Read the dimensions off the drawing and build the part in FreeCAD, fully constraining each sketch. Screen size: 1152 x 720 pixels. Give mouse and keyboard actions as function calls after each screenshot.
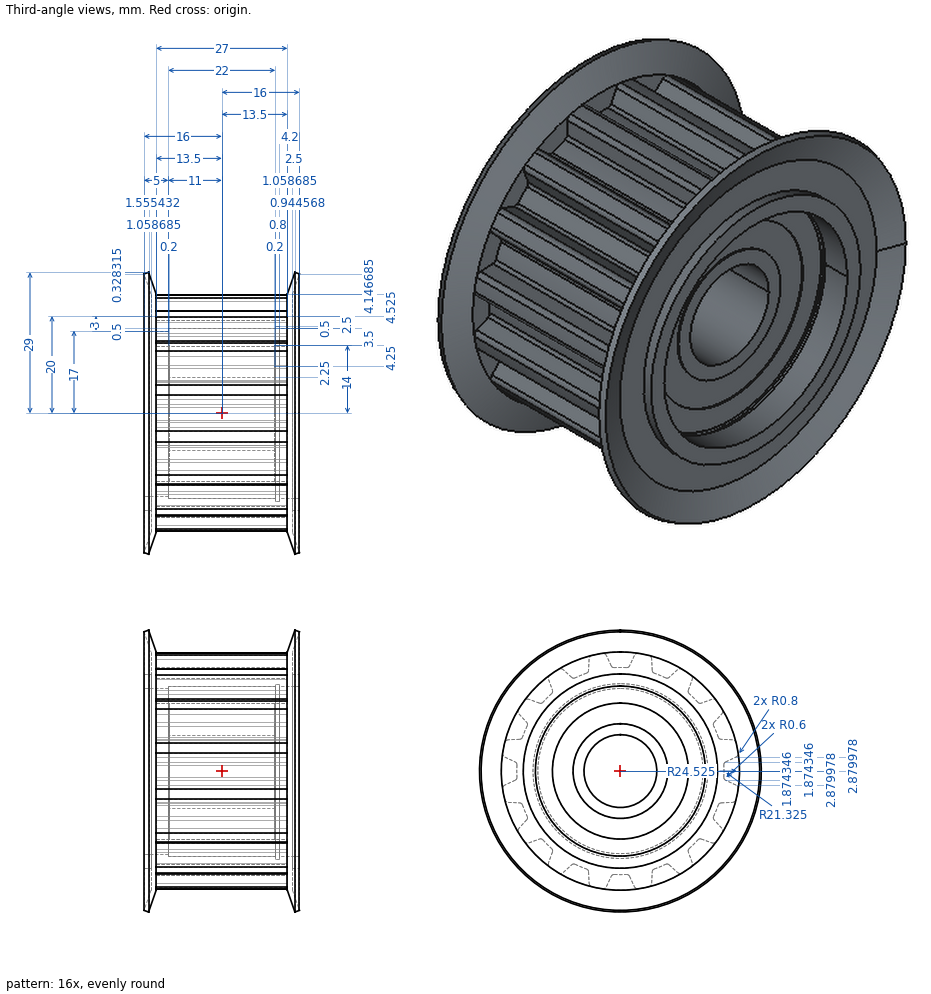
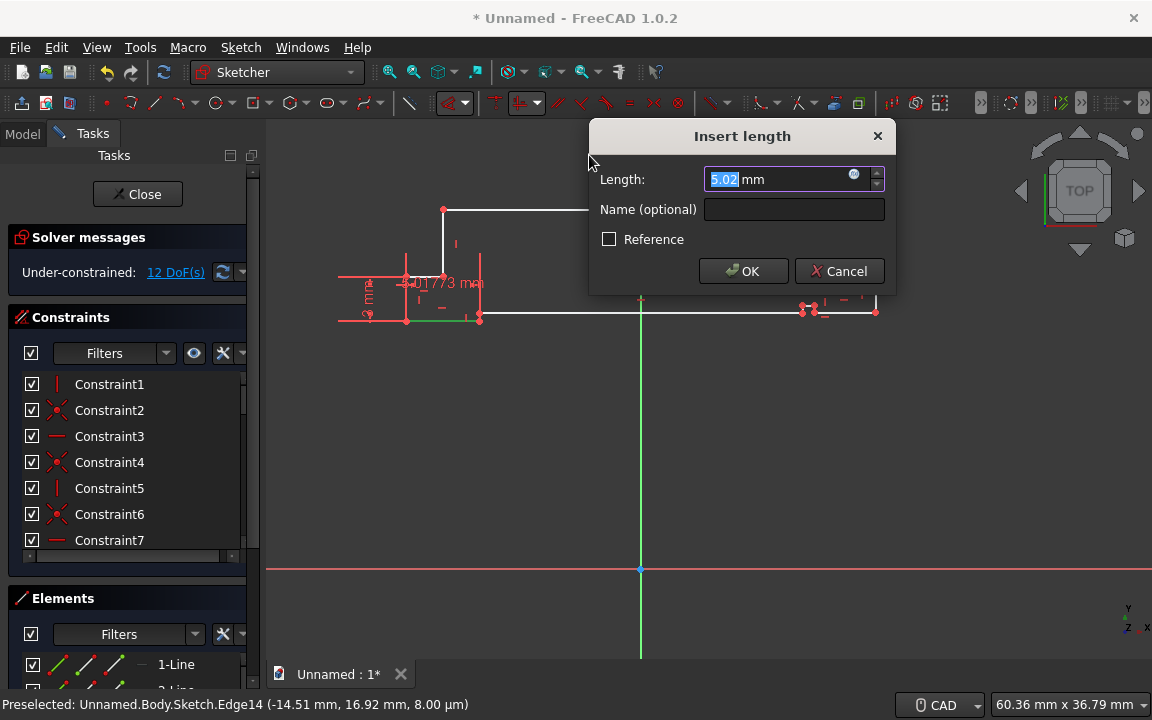
text(5)
key(Return)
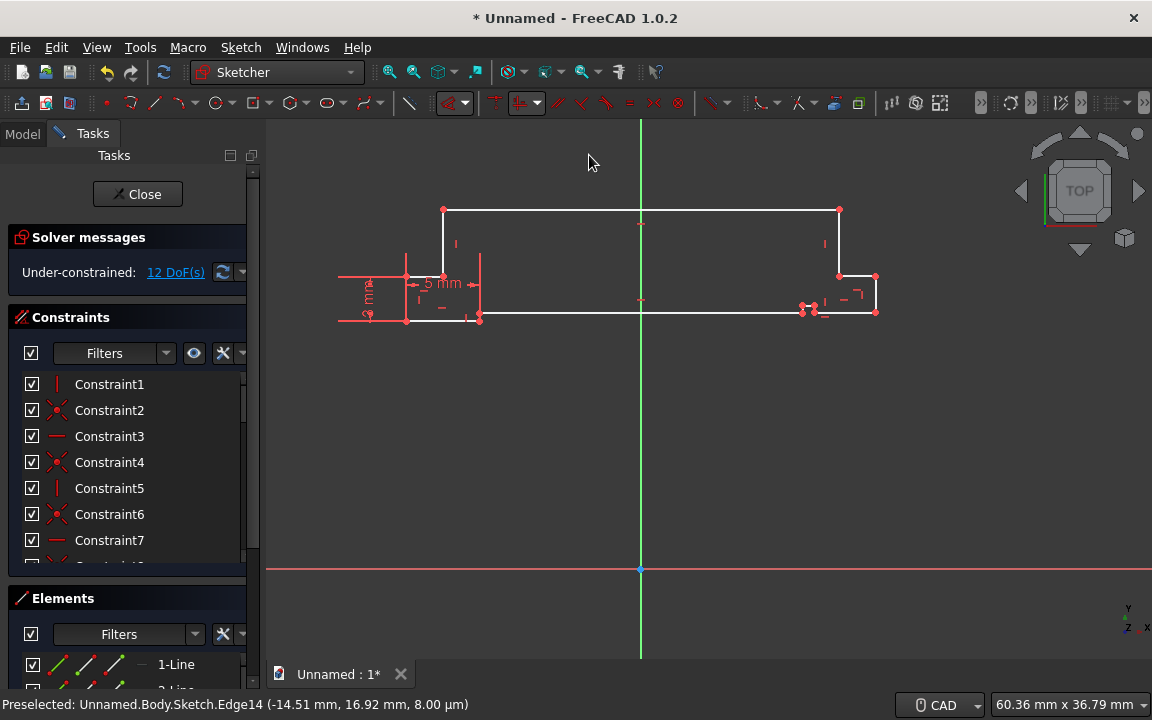
click(577, 313)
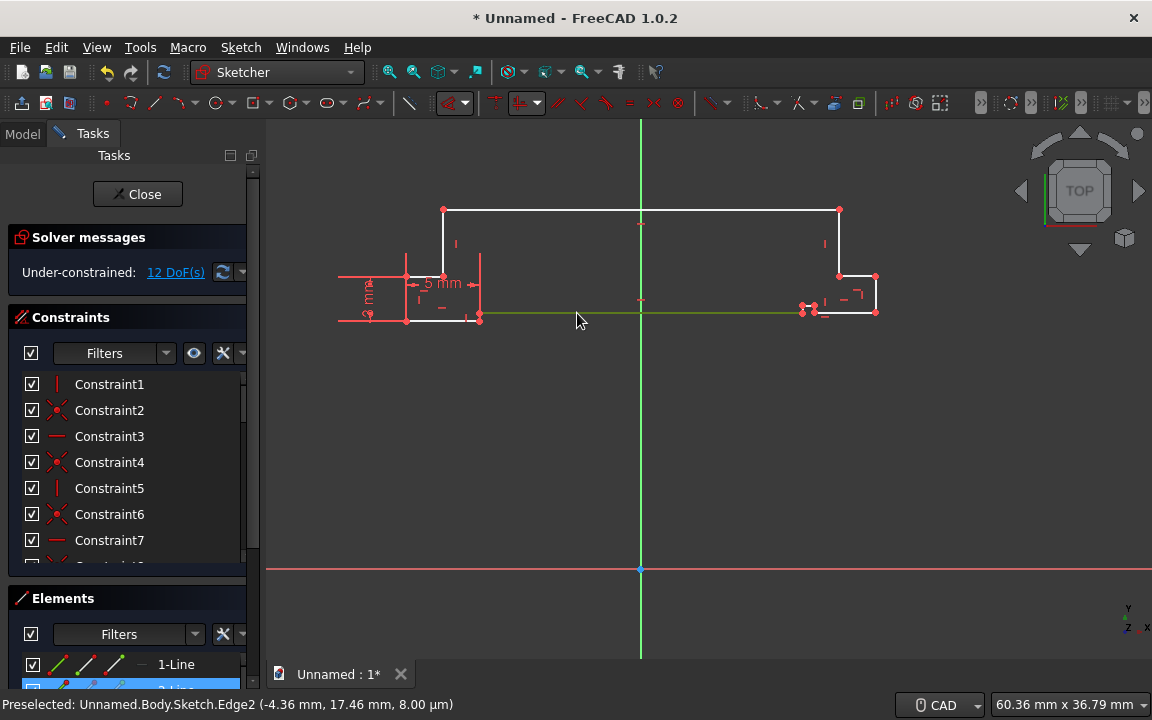
key(l)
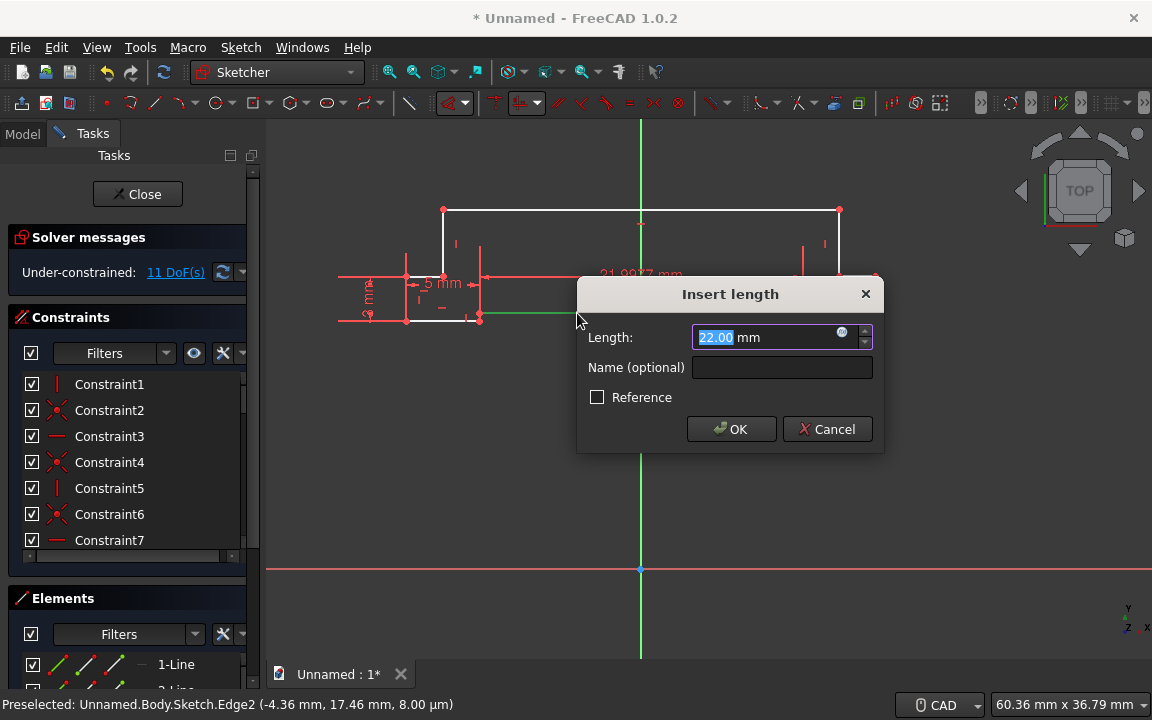
text(22)
key(Return)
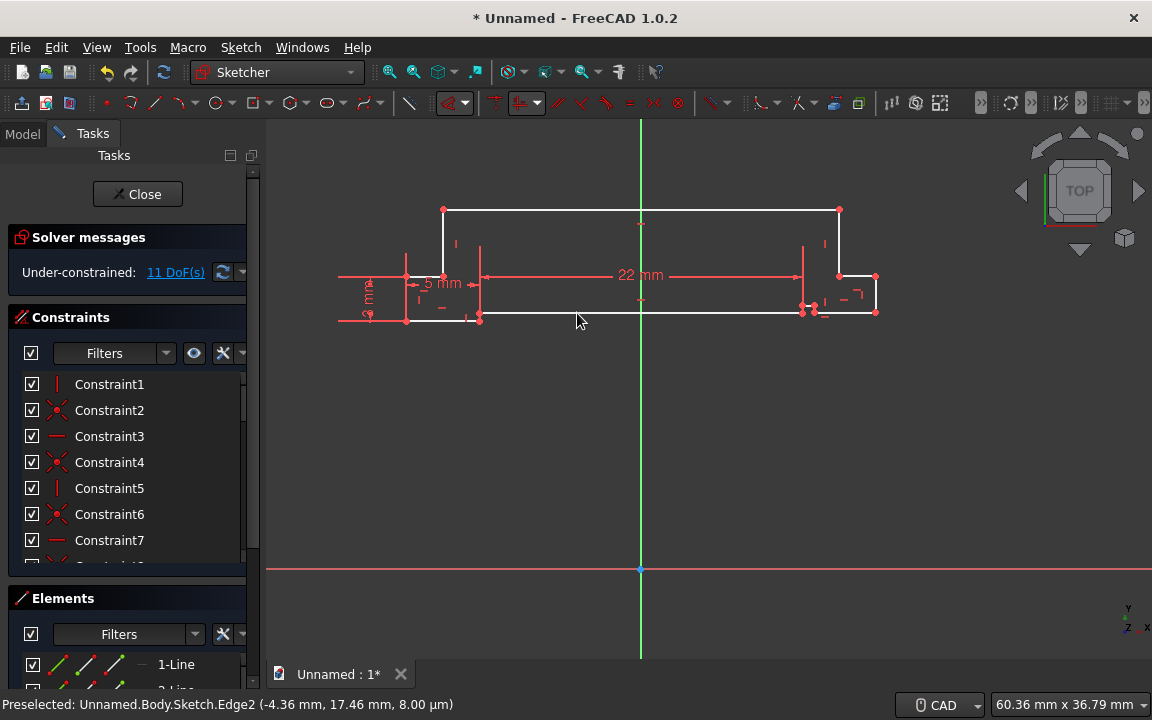
click(720, 210)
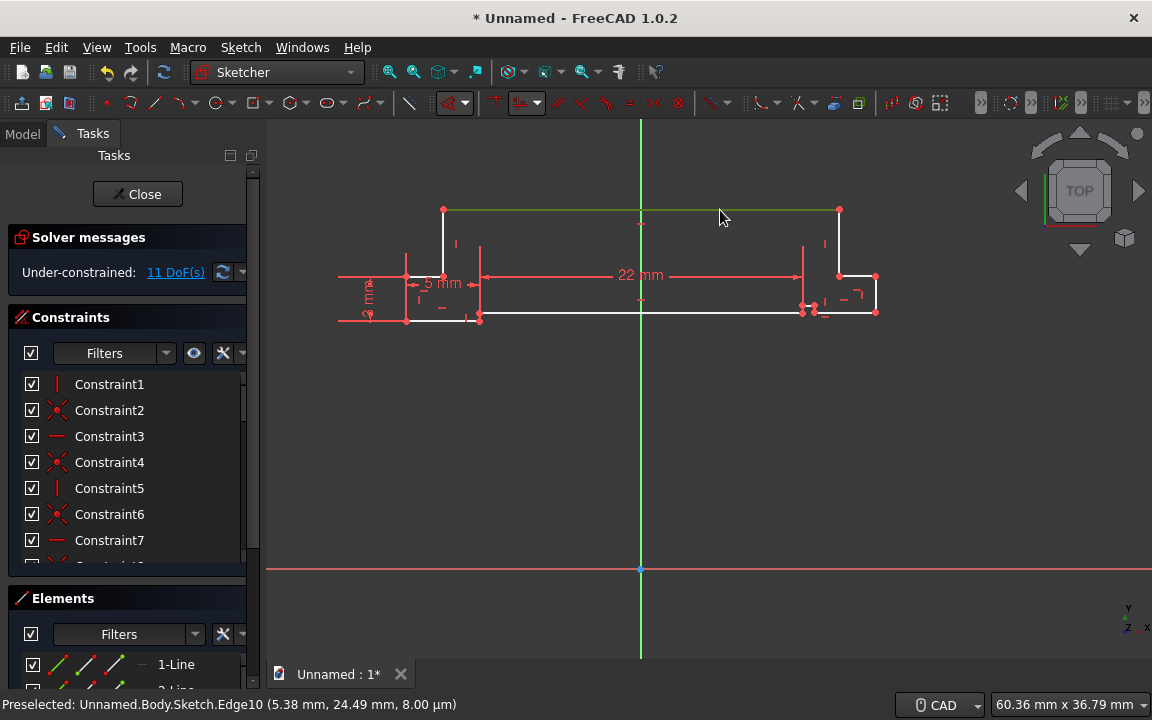
key(l)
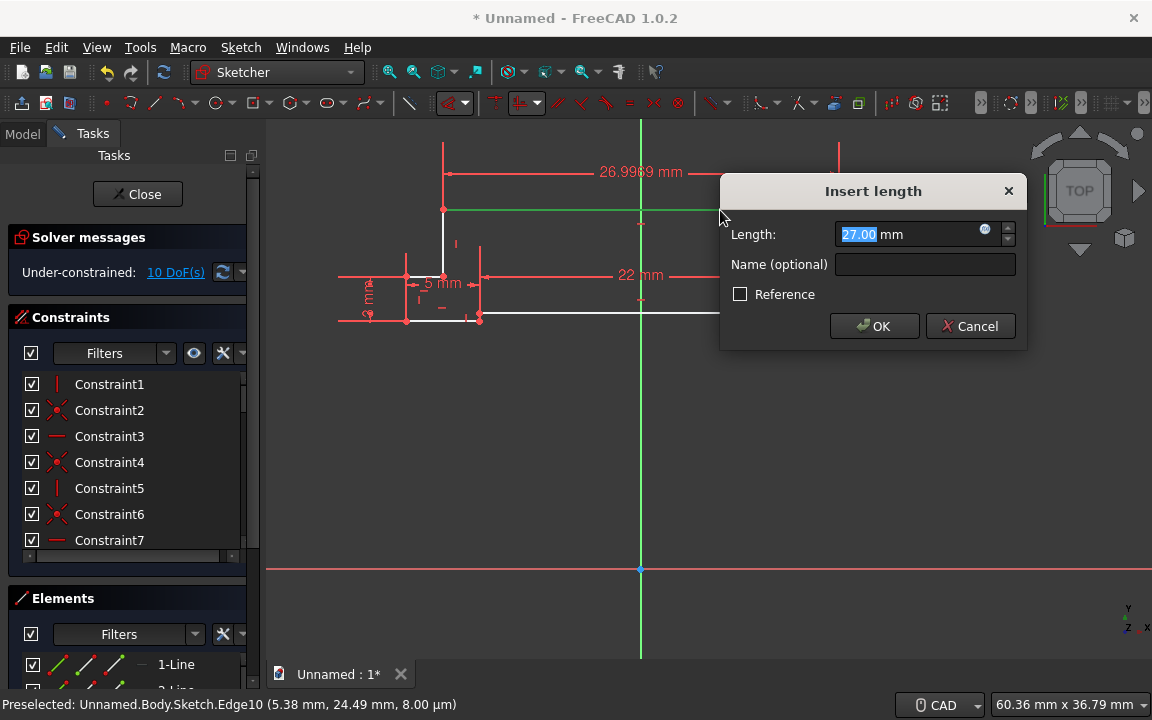
text(27)
key(Return)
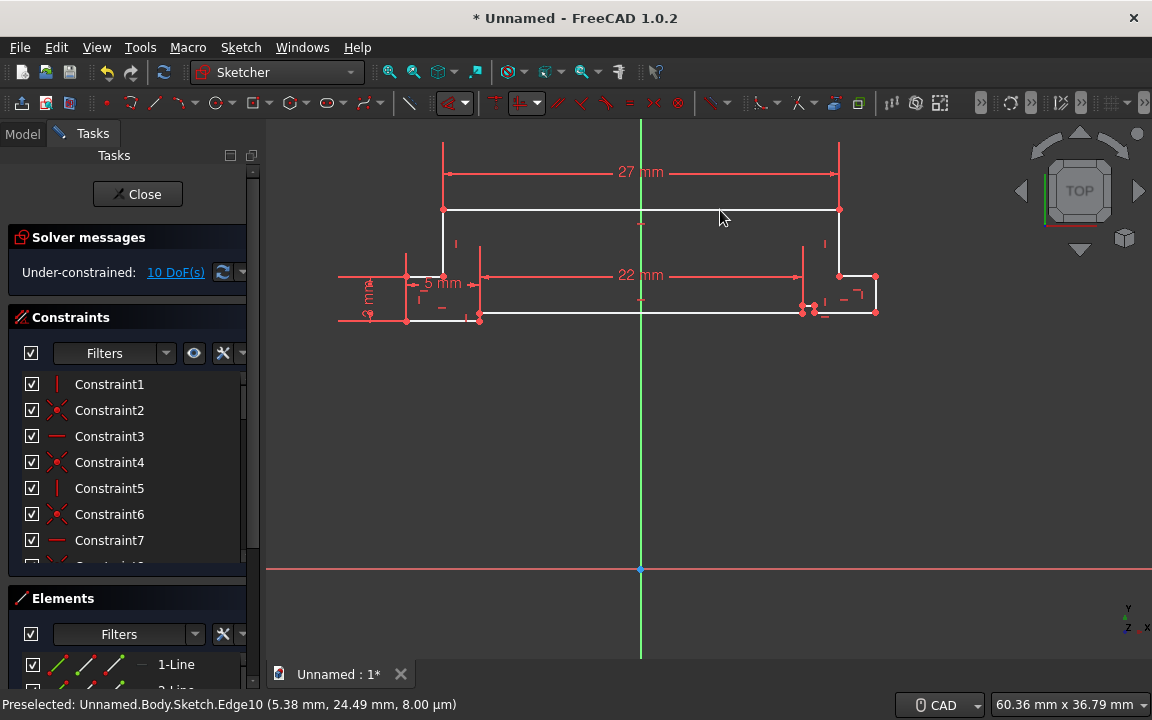
scroll(480, 317, up, 9)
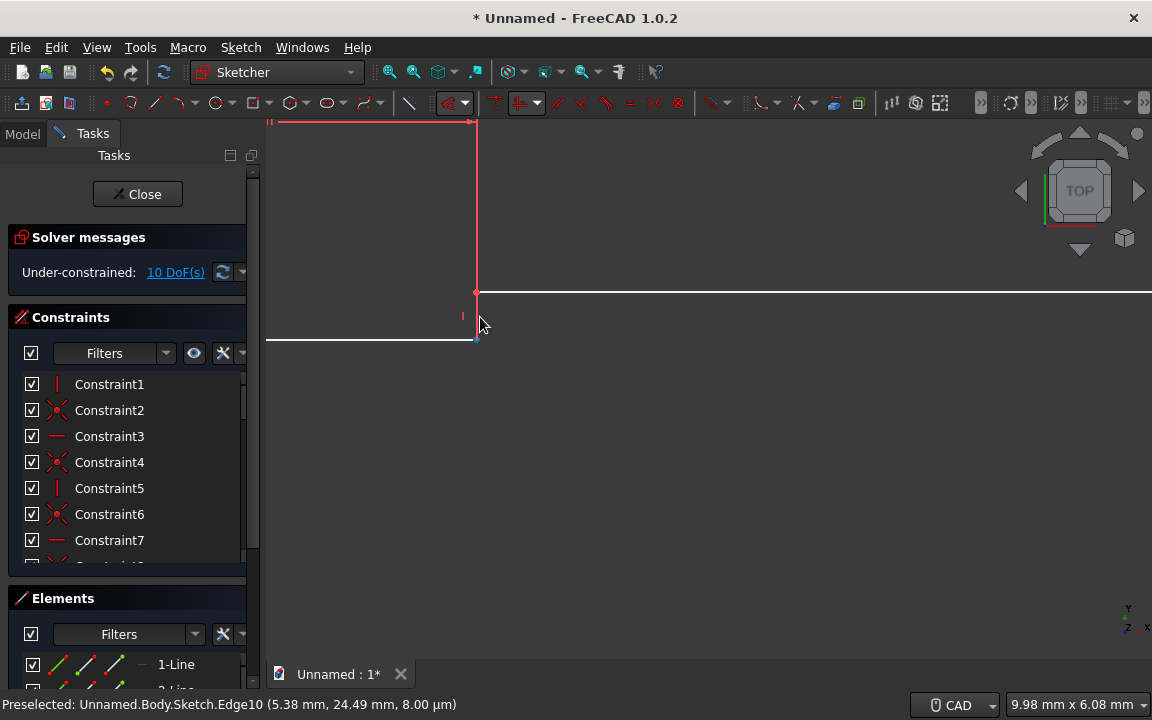
click(477, 316)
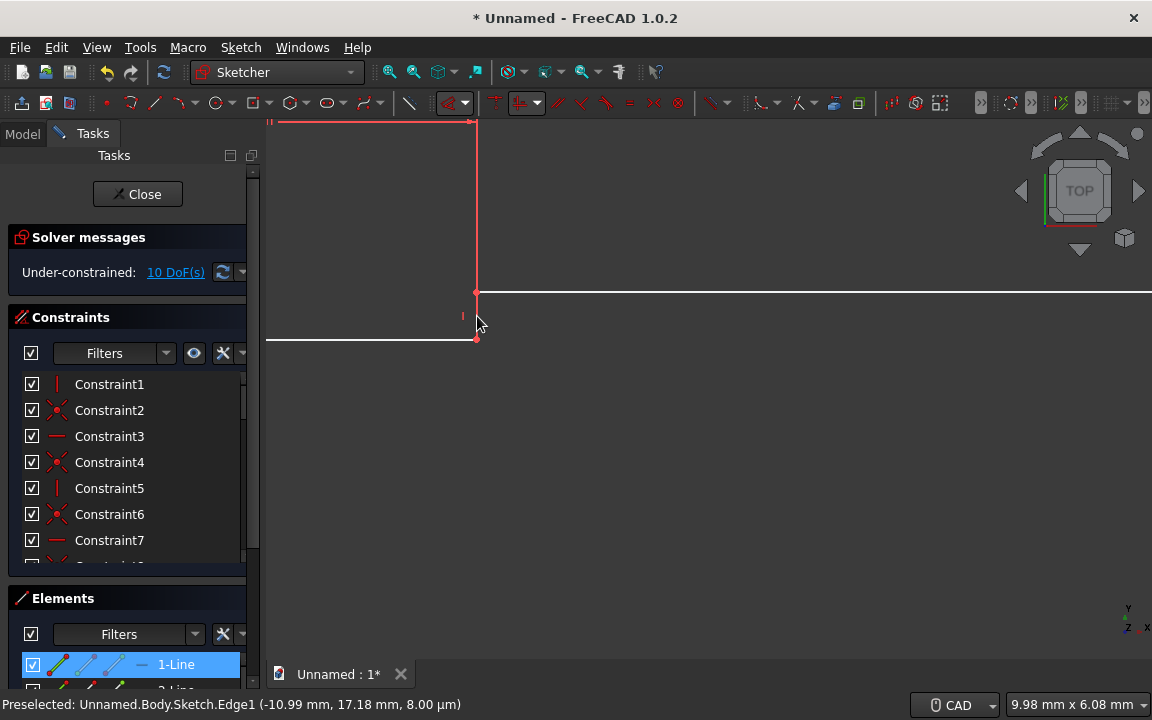
key(i)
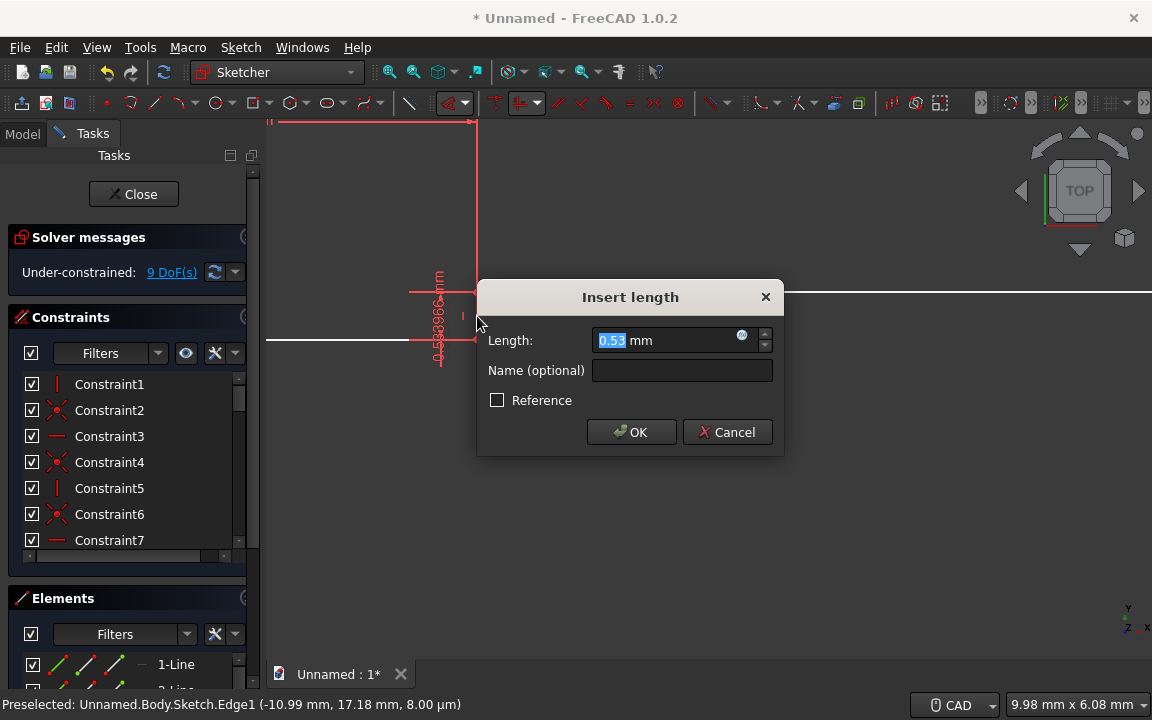
text(0.5)
key(Return)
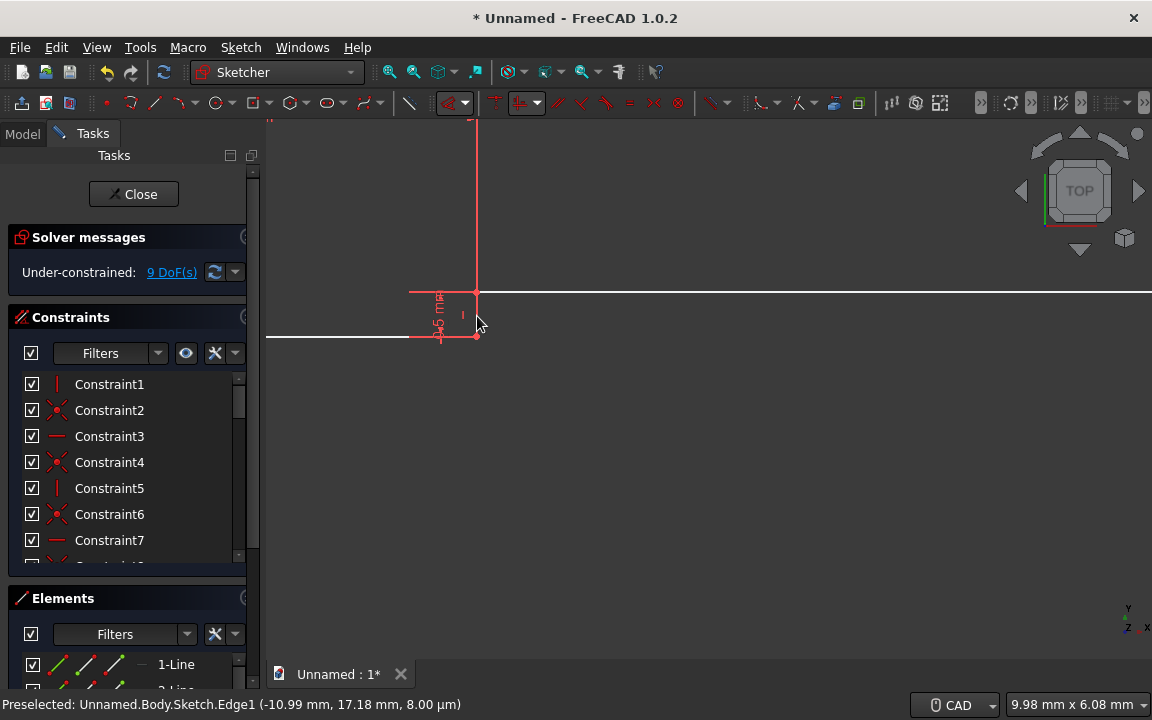
scroll(480, 317, down, 9)